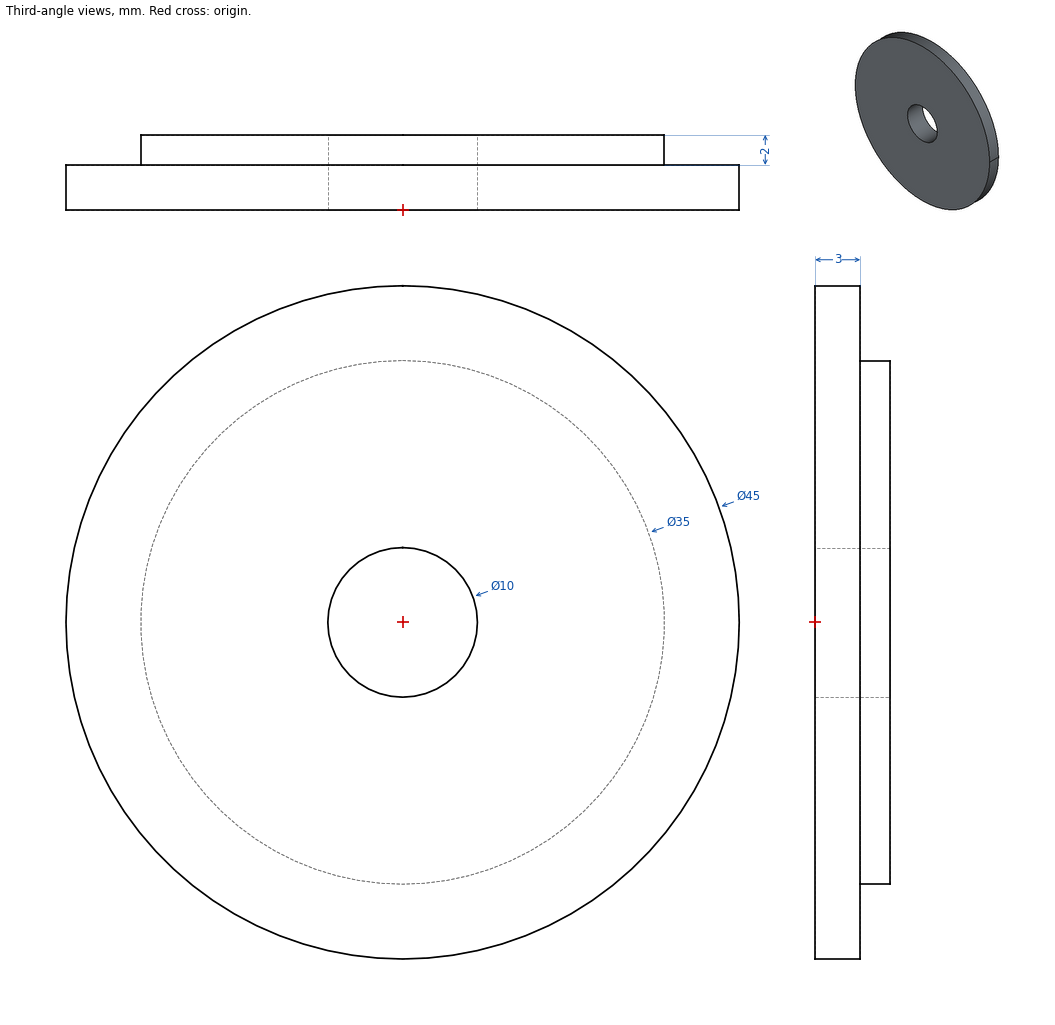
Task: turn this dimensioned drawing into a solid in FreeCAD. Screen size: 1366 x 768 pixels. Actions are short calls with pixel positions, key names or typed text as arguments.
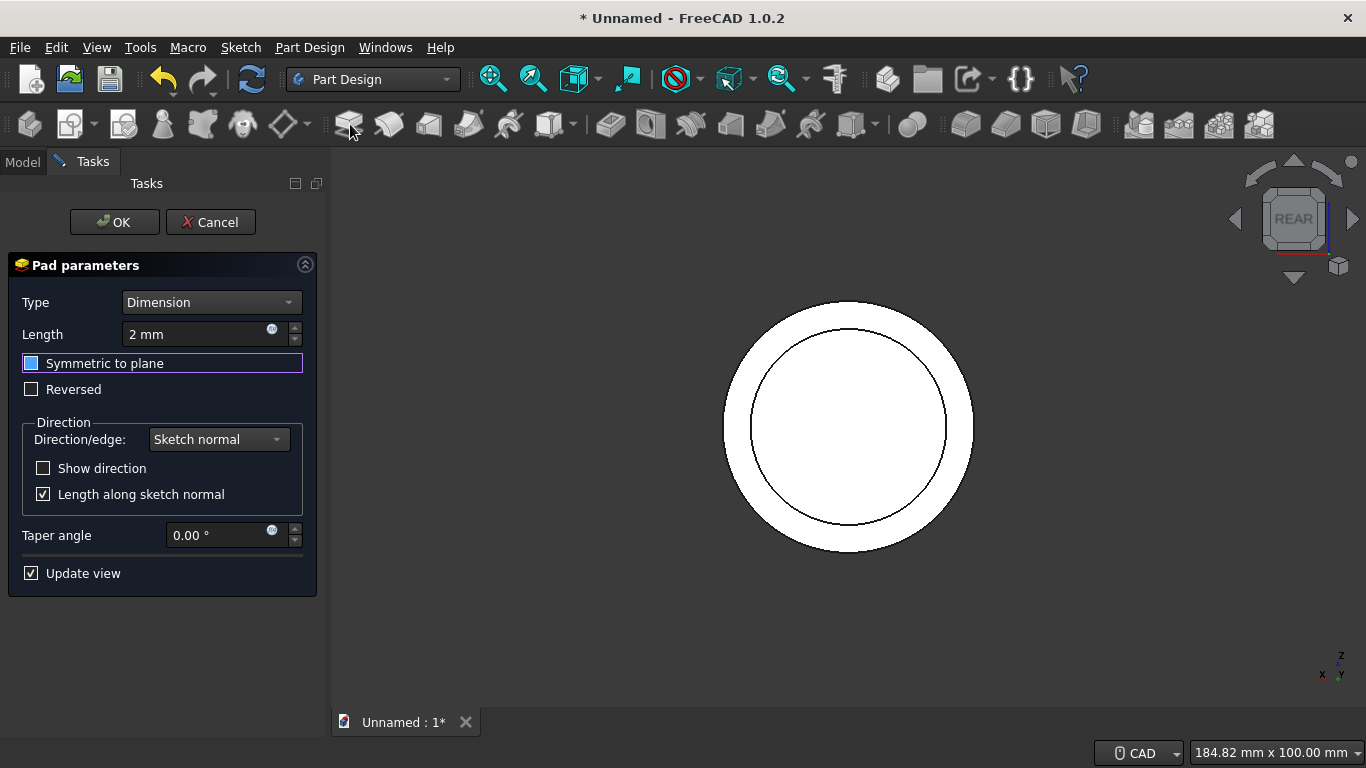
click(115, 222)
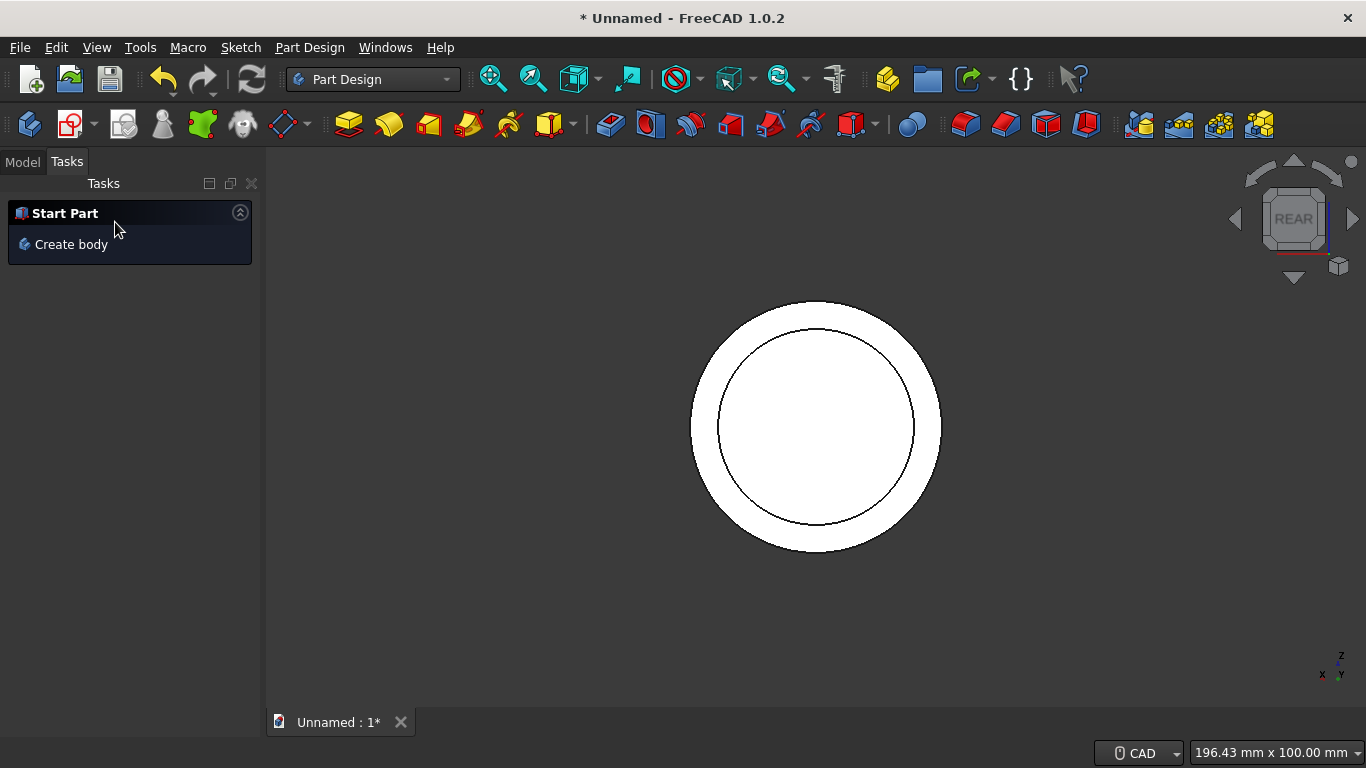
click(816, 426)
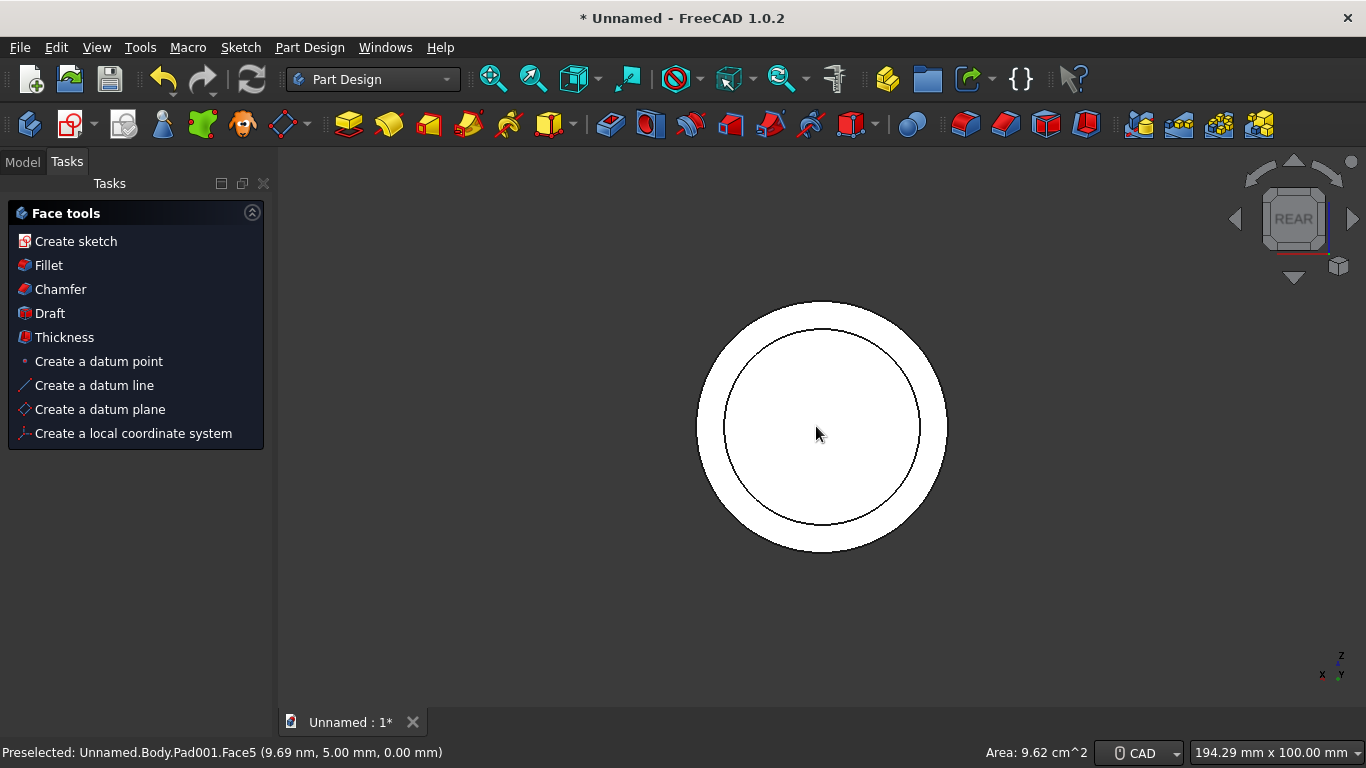
click(70, 124)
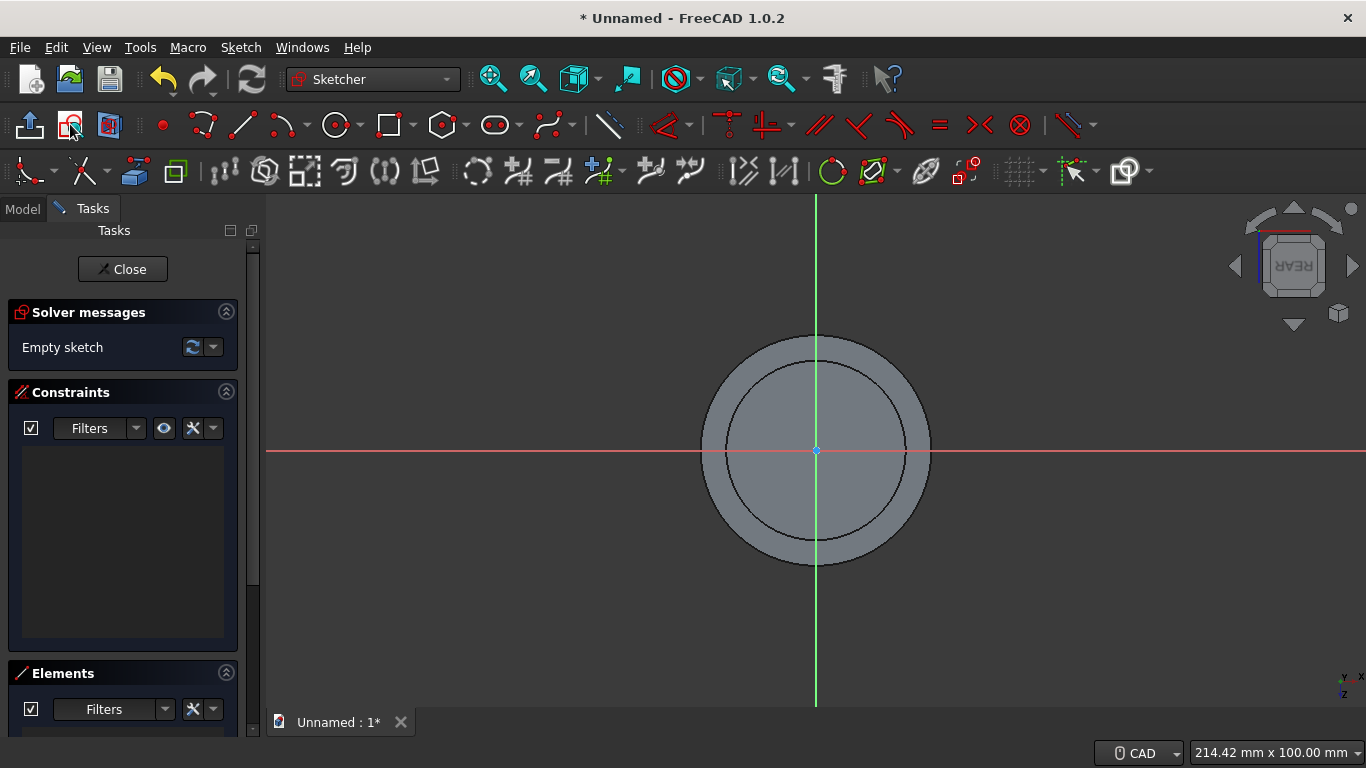
scroll(830, 450, up, 9)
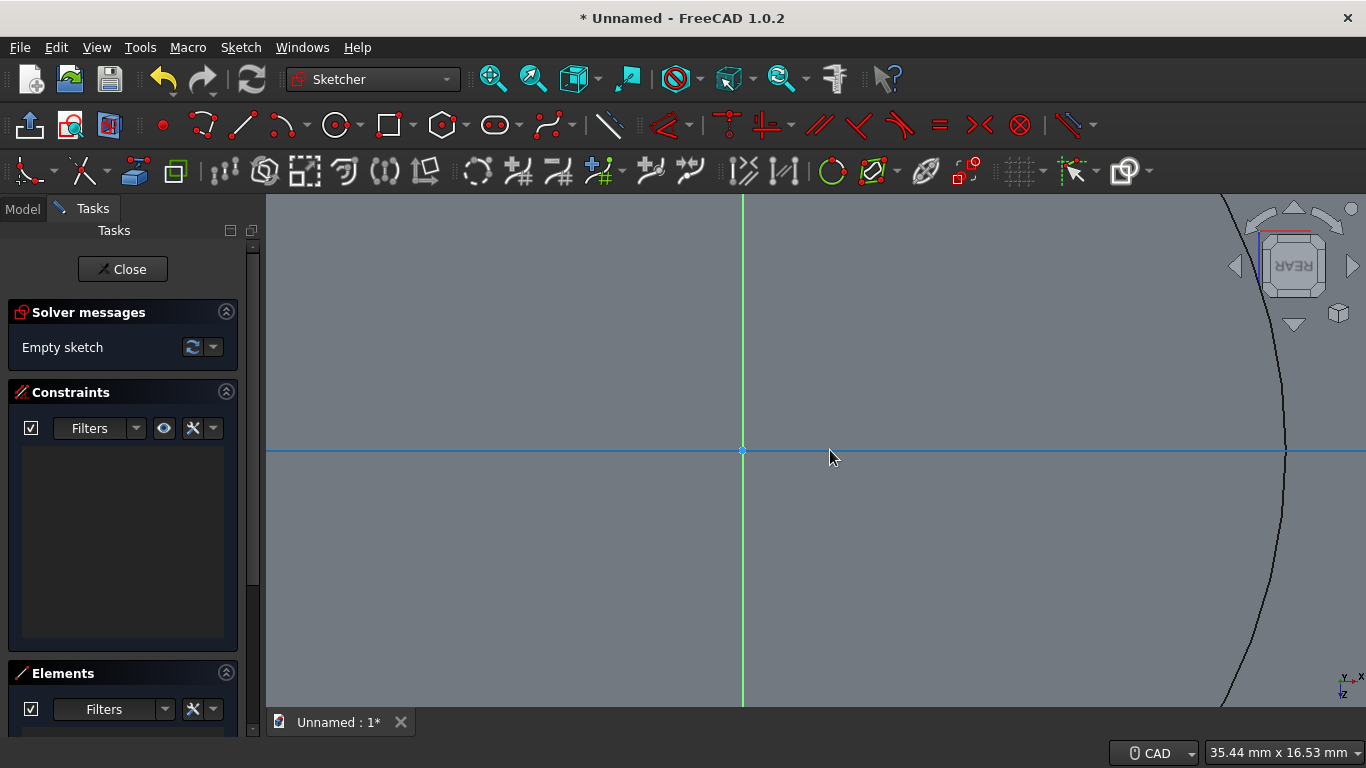
key(g)
key(c)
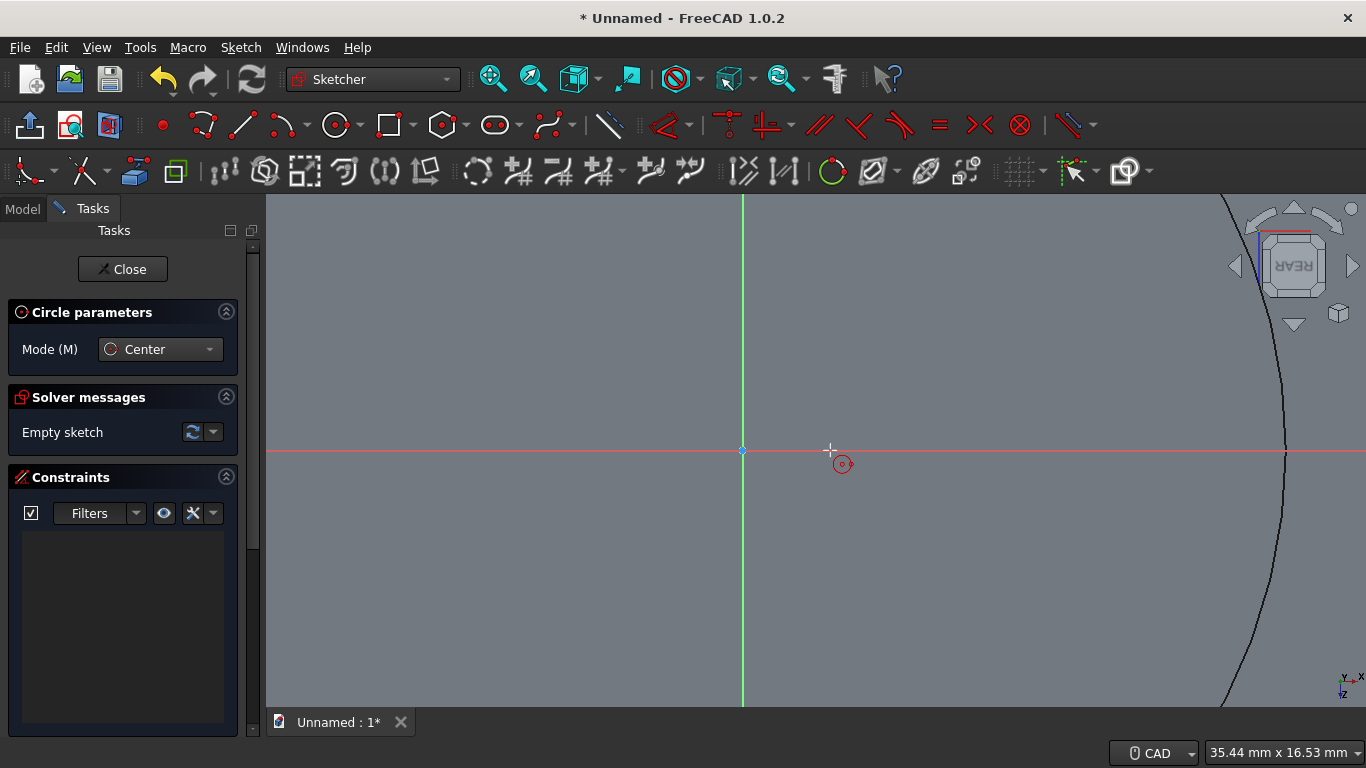
click(743, 450)
click(852, 341)
key(Escape)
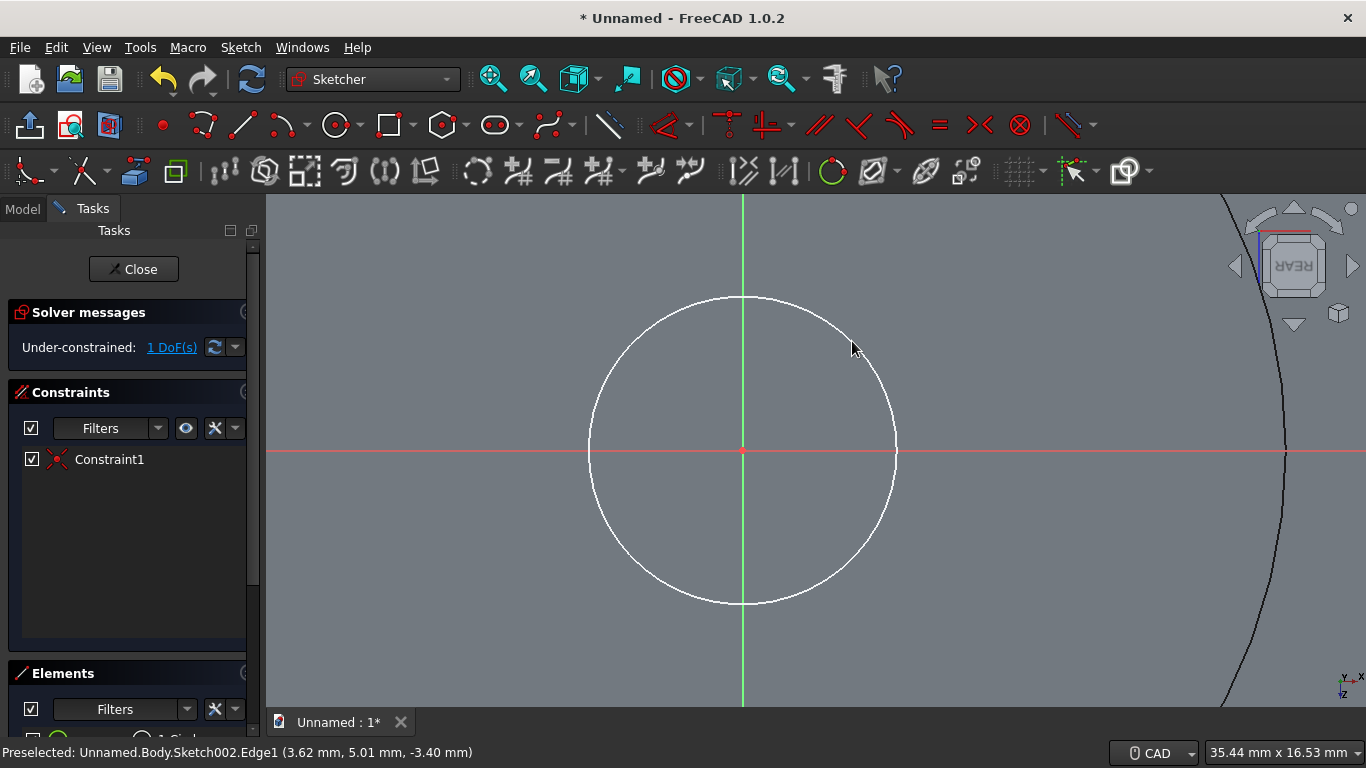
key(d)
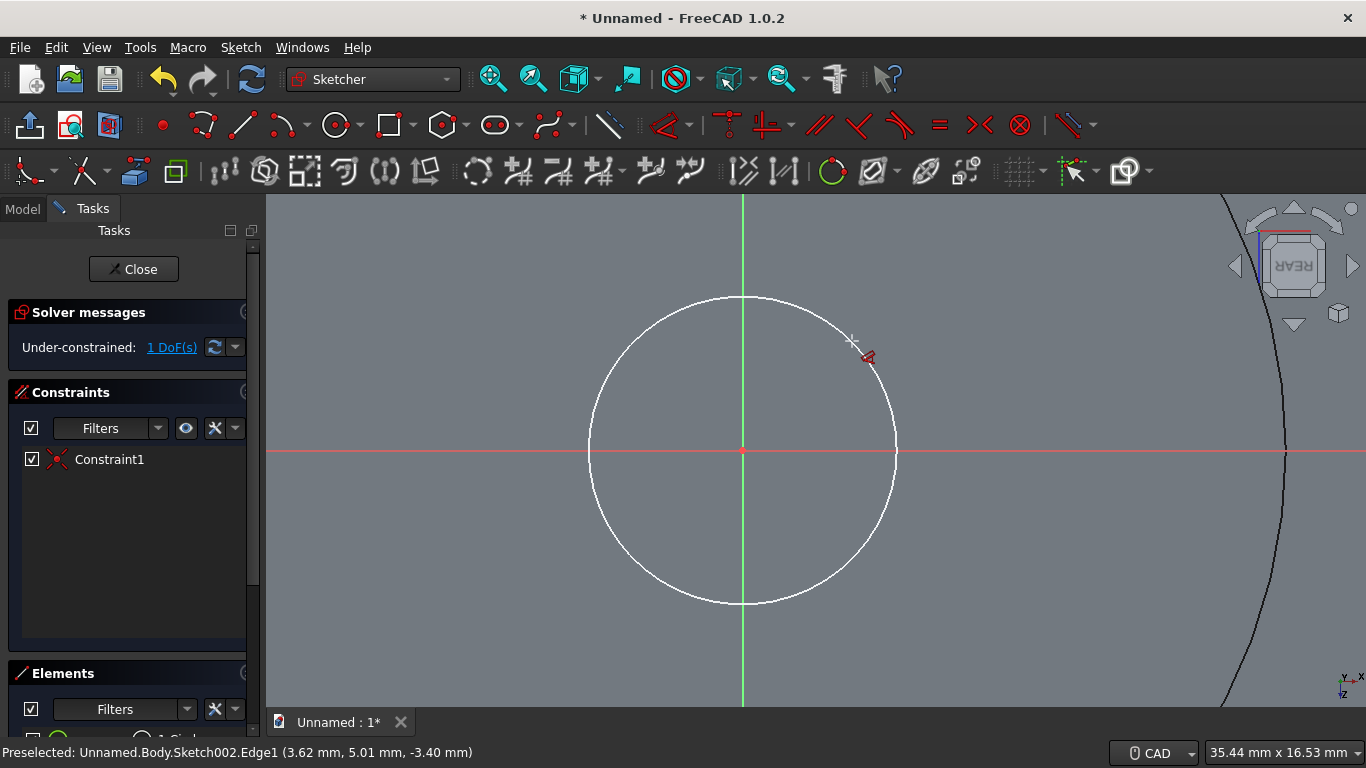
click(851, 341)
click(874, 318)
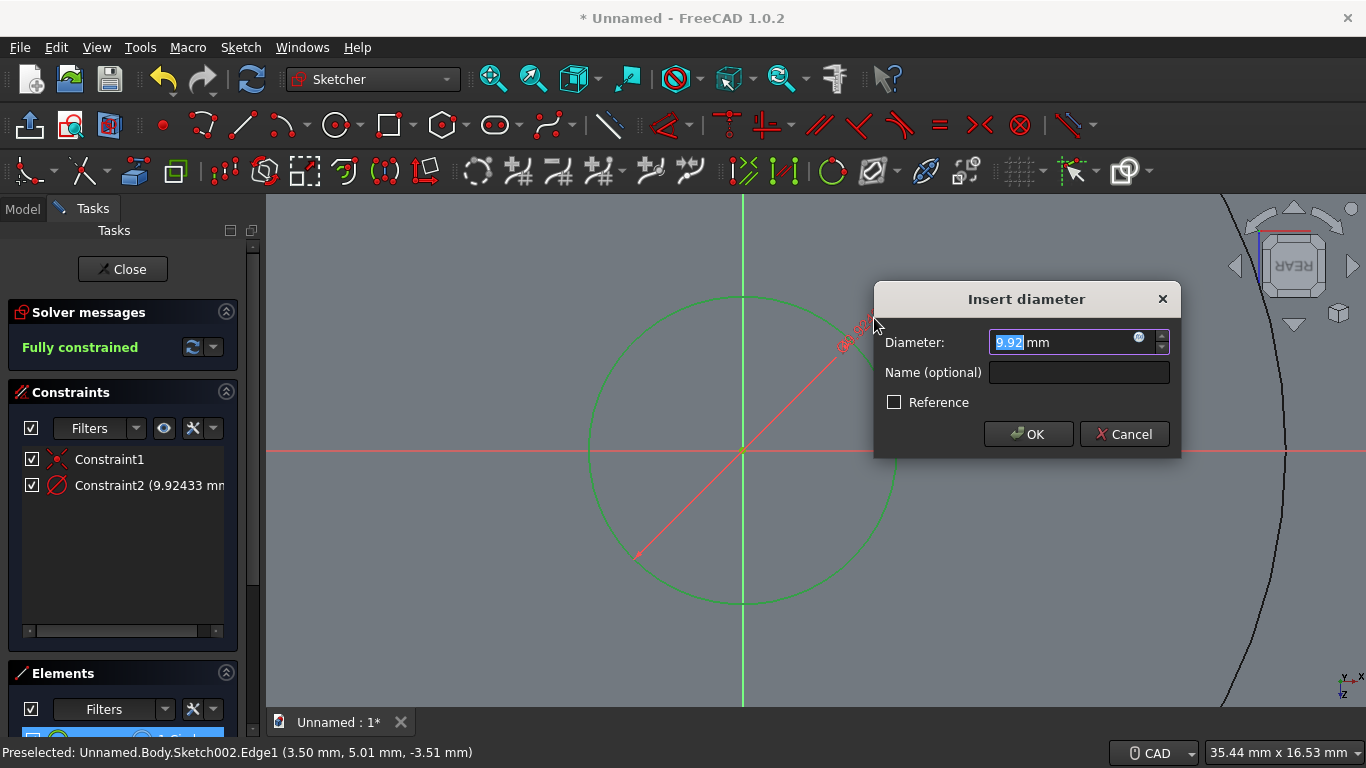
text(10)
key(Return)
key(Escape)